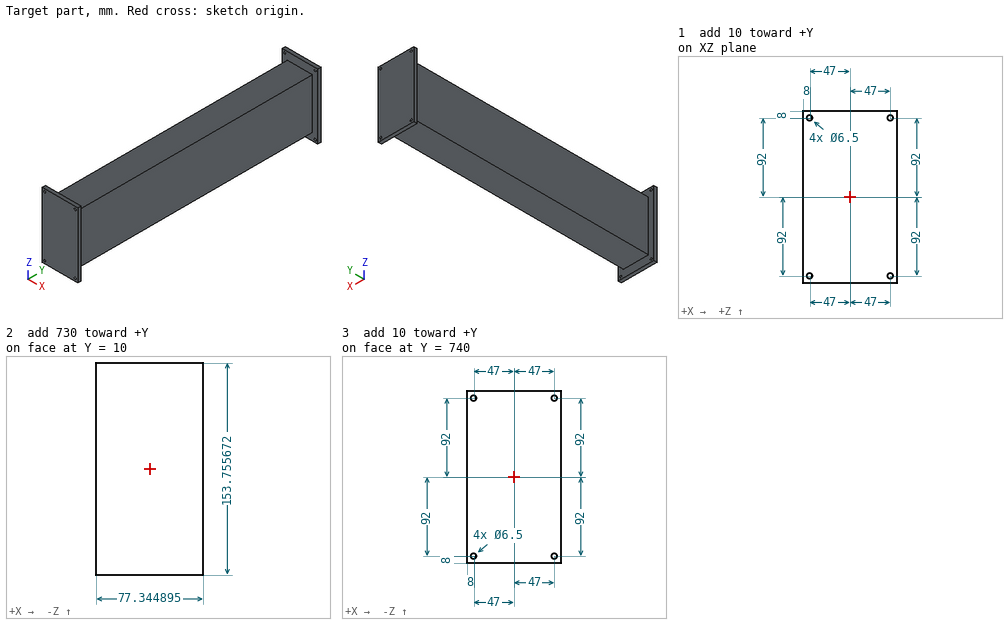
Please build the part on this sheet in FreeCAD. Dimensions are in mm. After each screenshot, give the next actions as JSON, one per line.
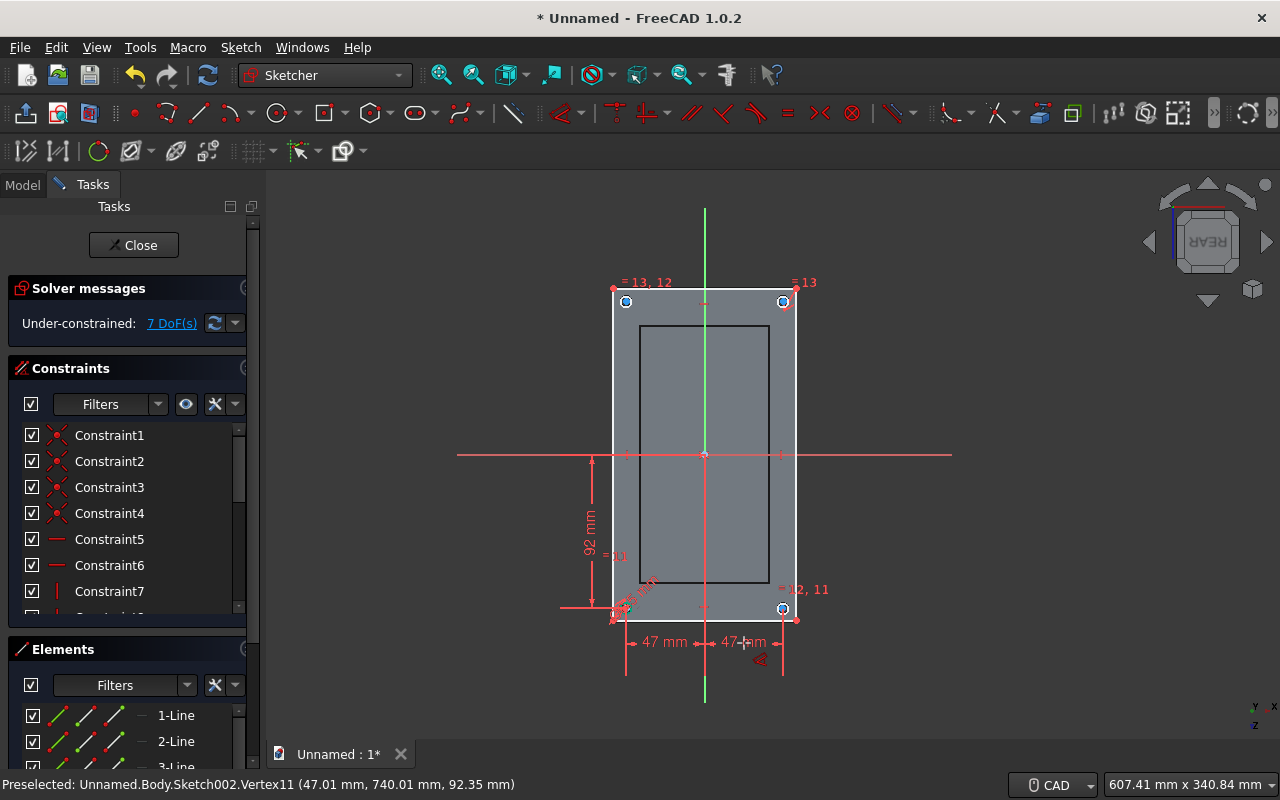
{"action": "left_click", "coordinate": [783, 609]}
{"action": "left_click", "coordinate": [817, 532]}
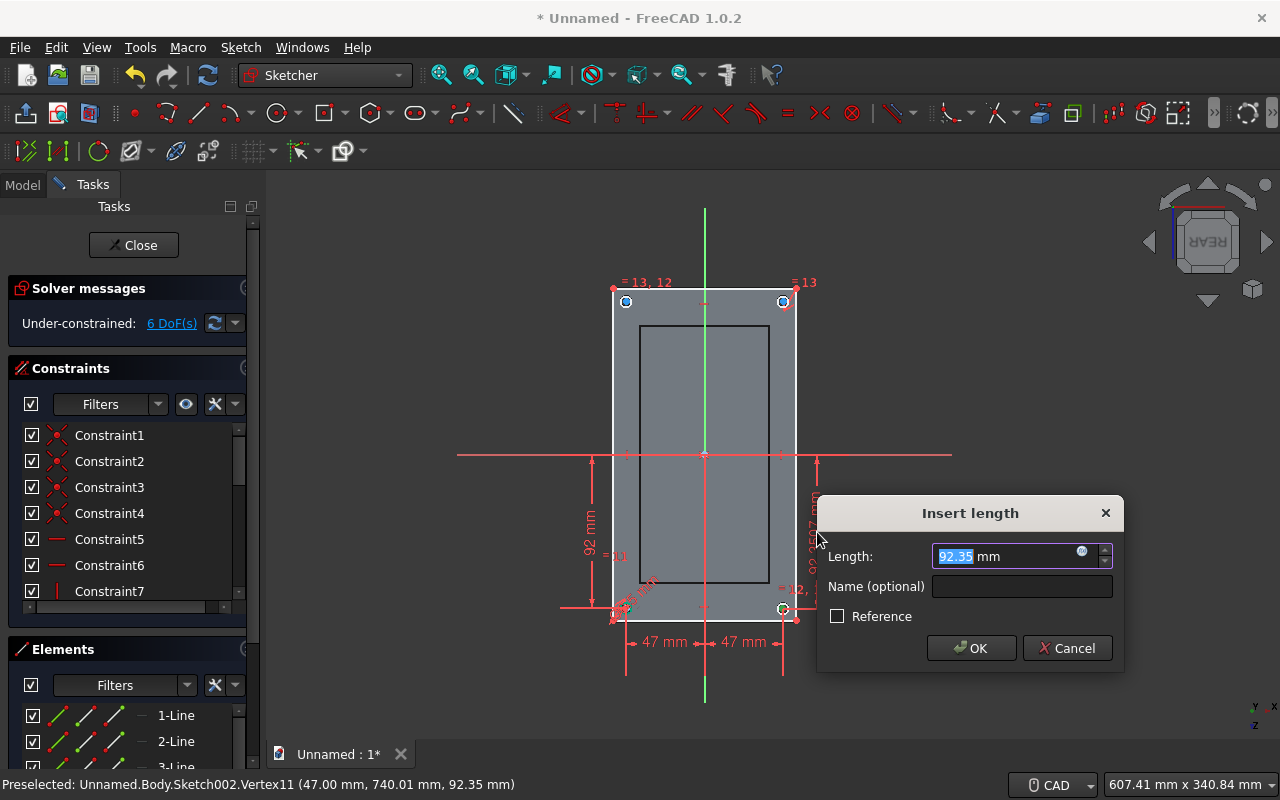
{"action": "type", "text": "92"}
{"action": "key", "text": "Return"}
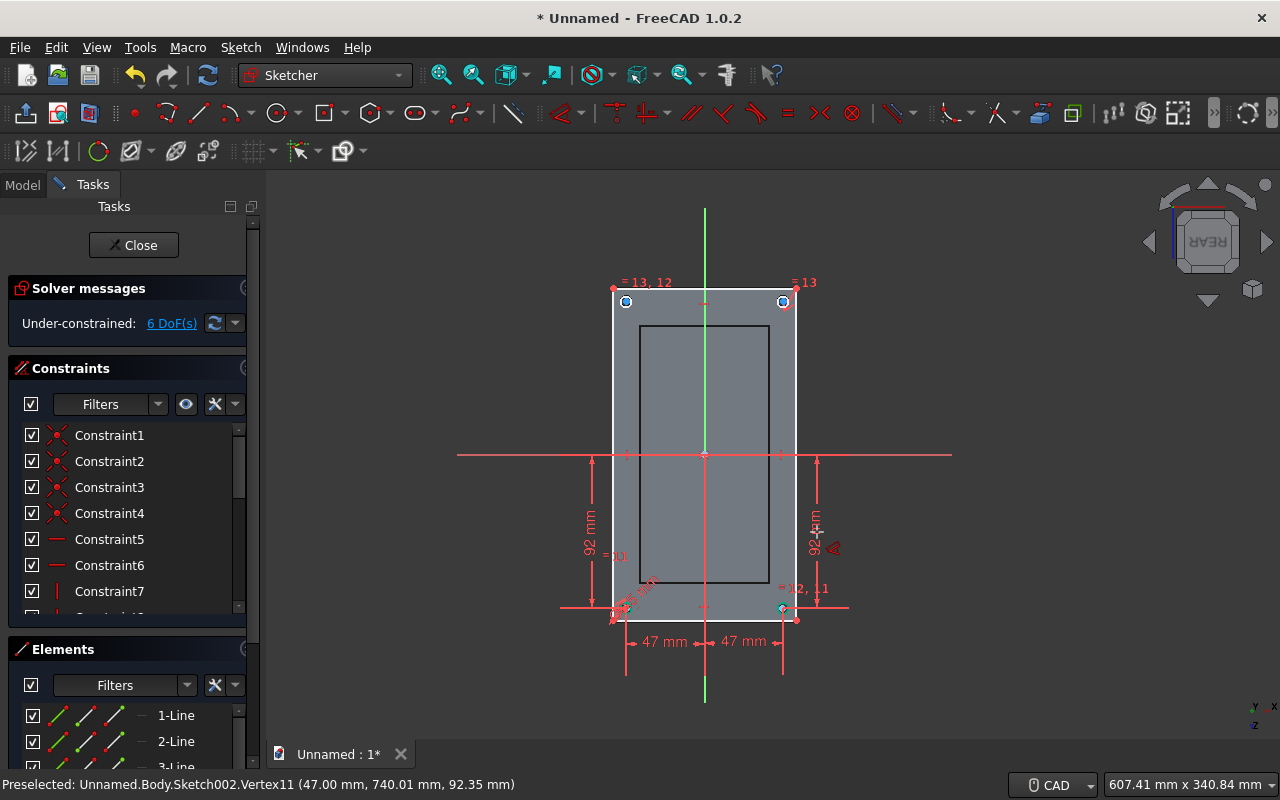
{"action": "left_click", "coordinate": [626, 302]}
{"action": "left_click", "coordinate": [665, 268]}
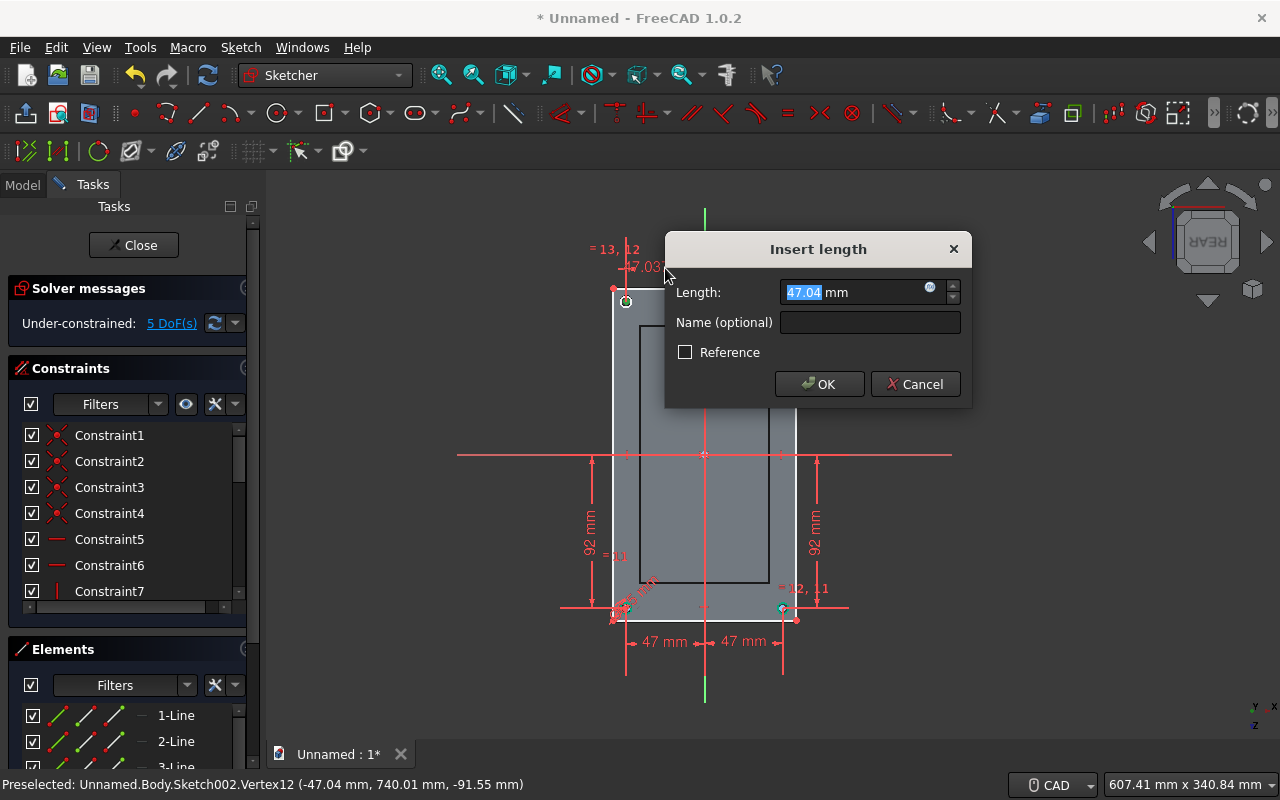
{"action": "type", "text": "47"}
{"action": "key", "text": "Return"}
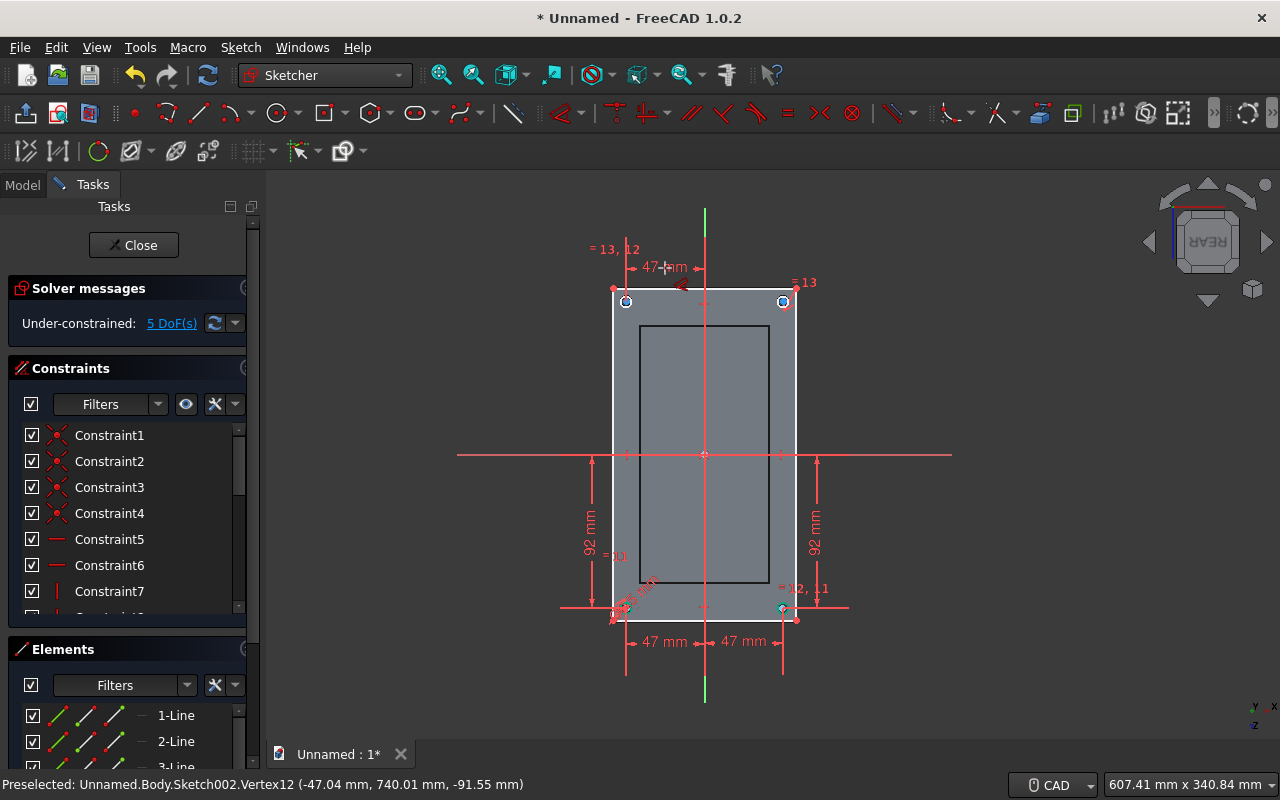
{"action": "left_click", "coordinate": [626, 302]}
{"action": "left_click", "coordinate": [592, 378]}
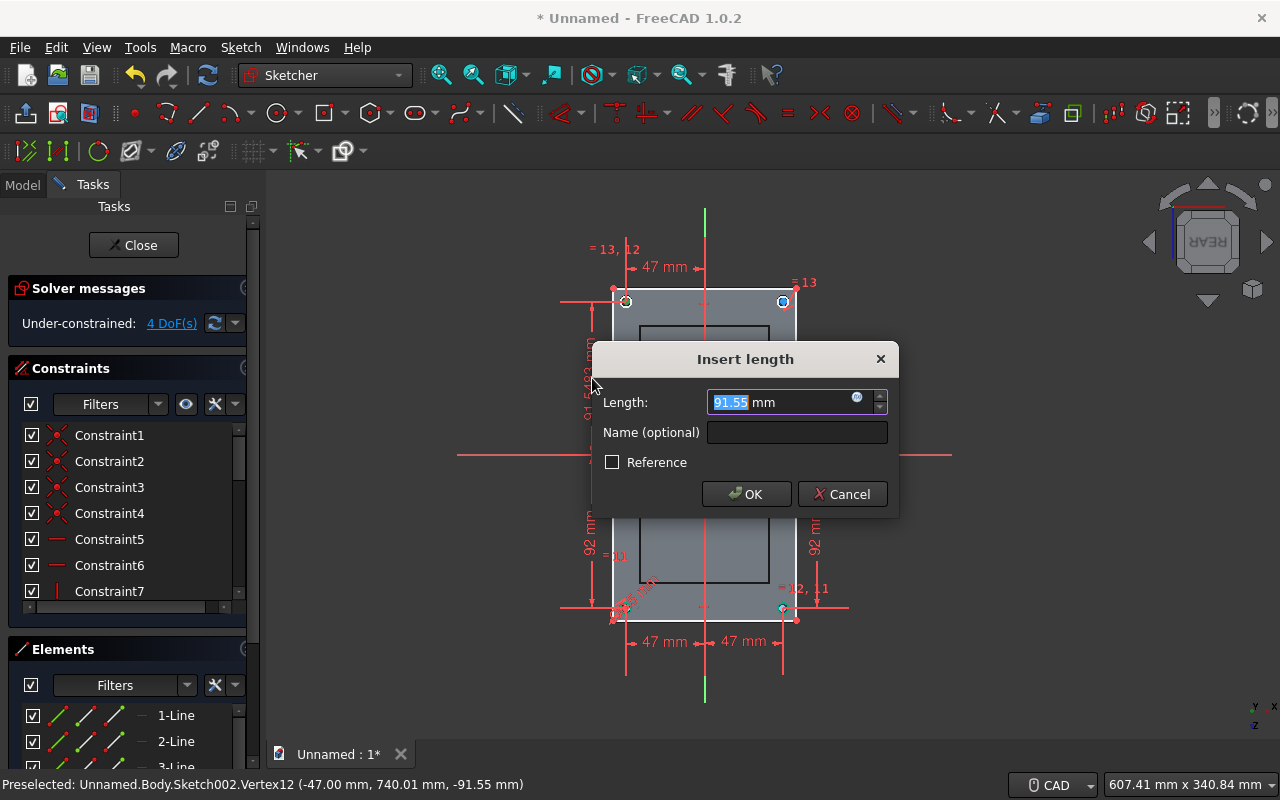
{"action": "type", "text": "92"}
{"action": "key", "text": "Return"}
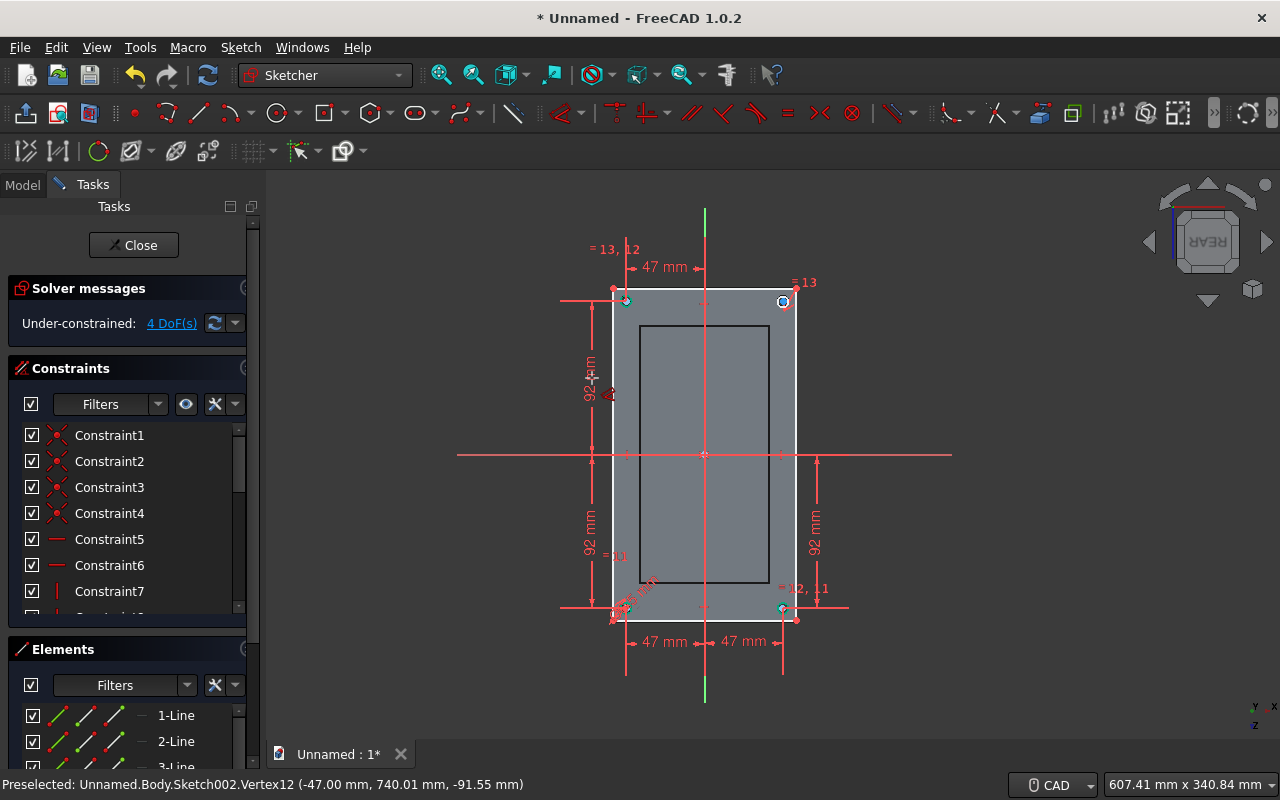
{"action": "left_click", "coordinate": [783, 302]}
{"action": "left_click", "coordinate": [744, 268]}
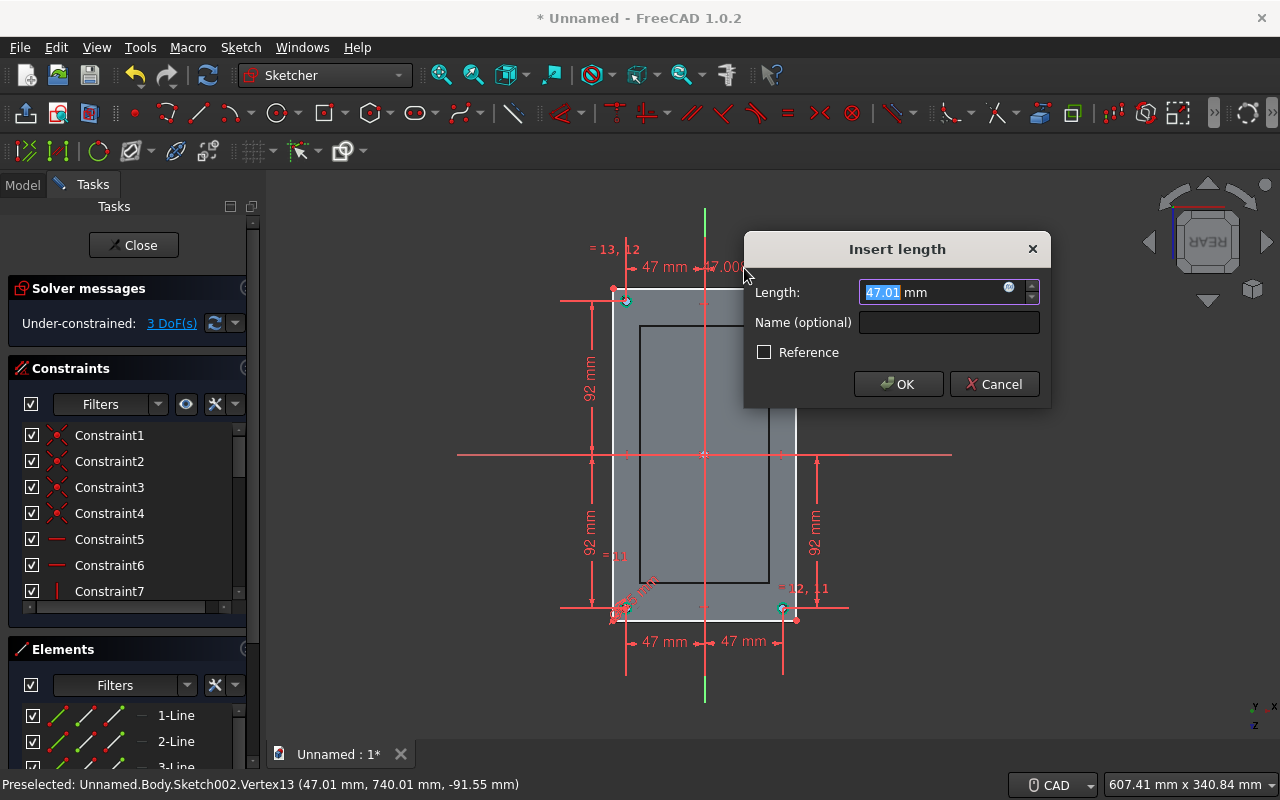
{"action": "type", "text": "47"}
{"action": "key", "text": "Return"}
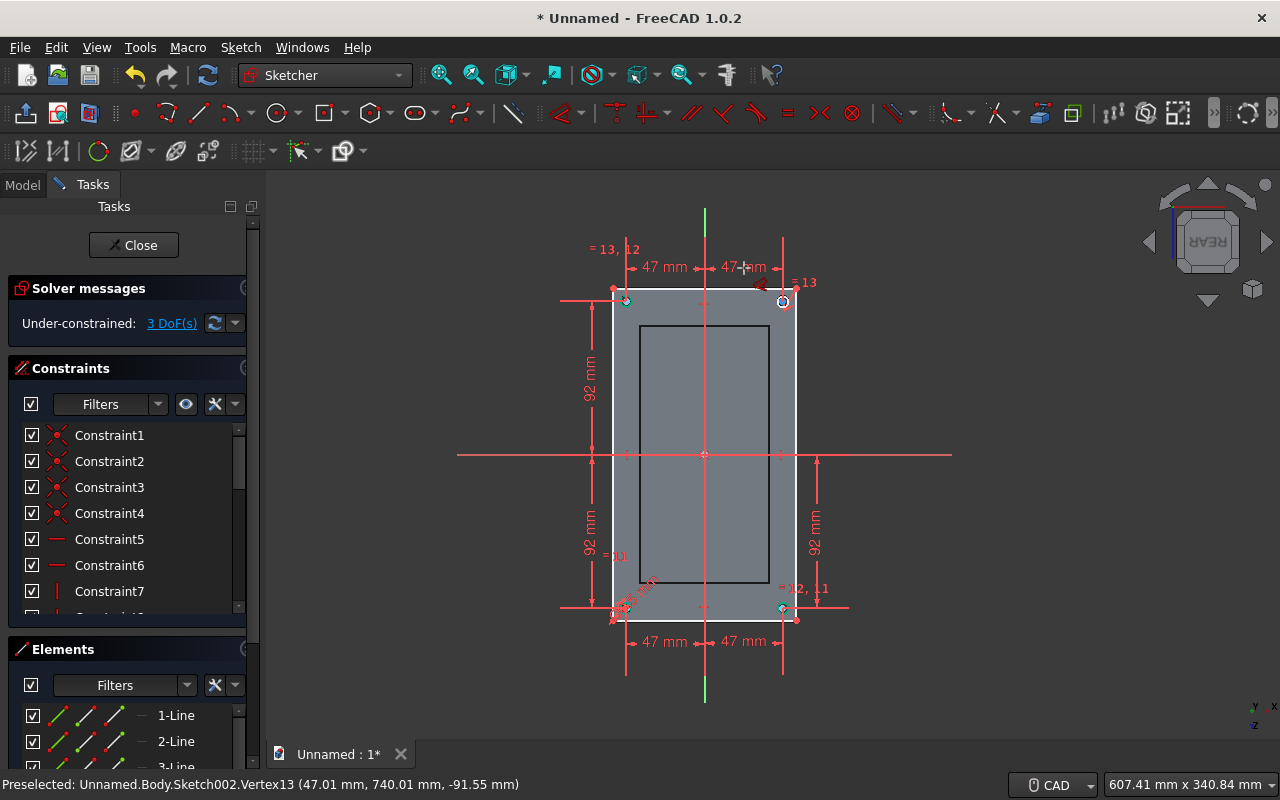
{"action": "left_click", "coordinate": [783, 302]}
{"action": "left_click", "coordinate": [817, 378]}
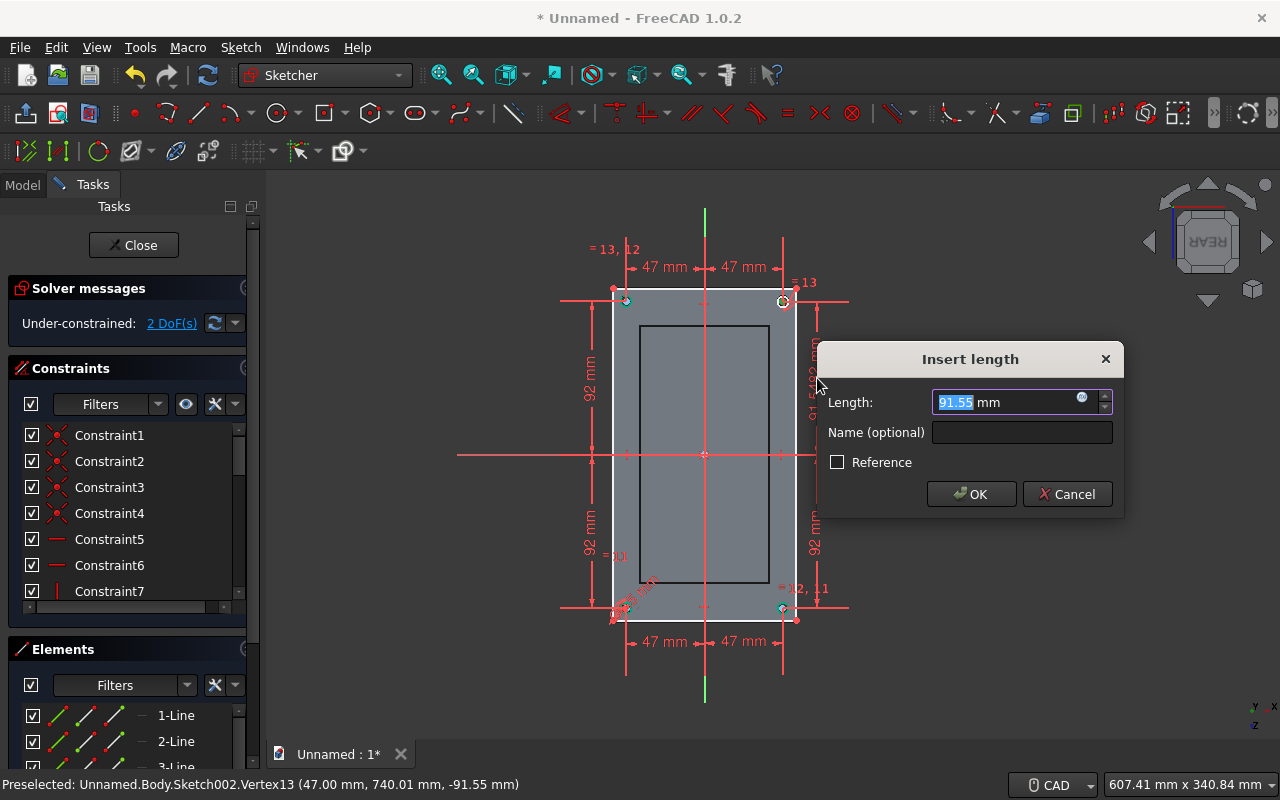
{"action": "type", "text": "92"}
{"action": "key", "text": "Return"}